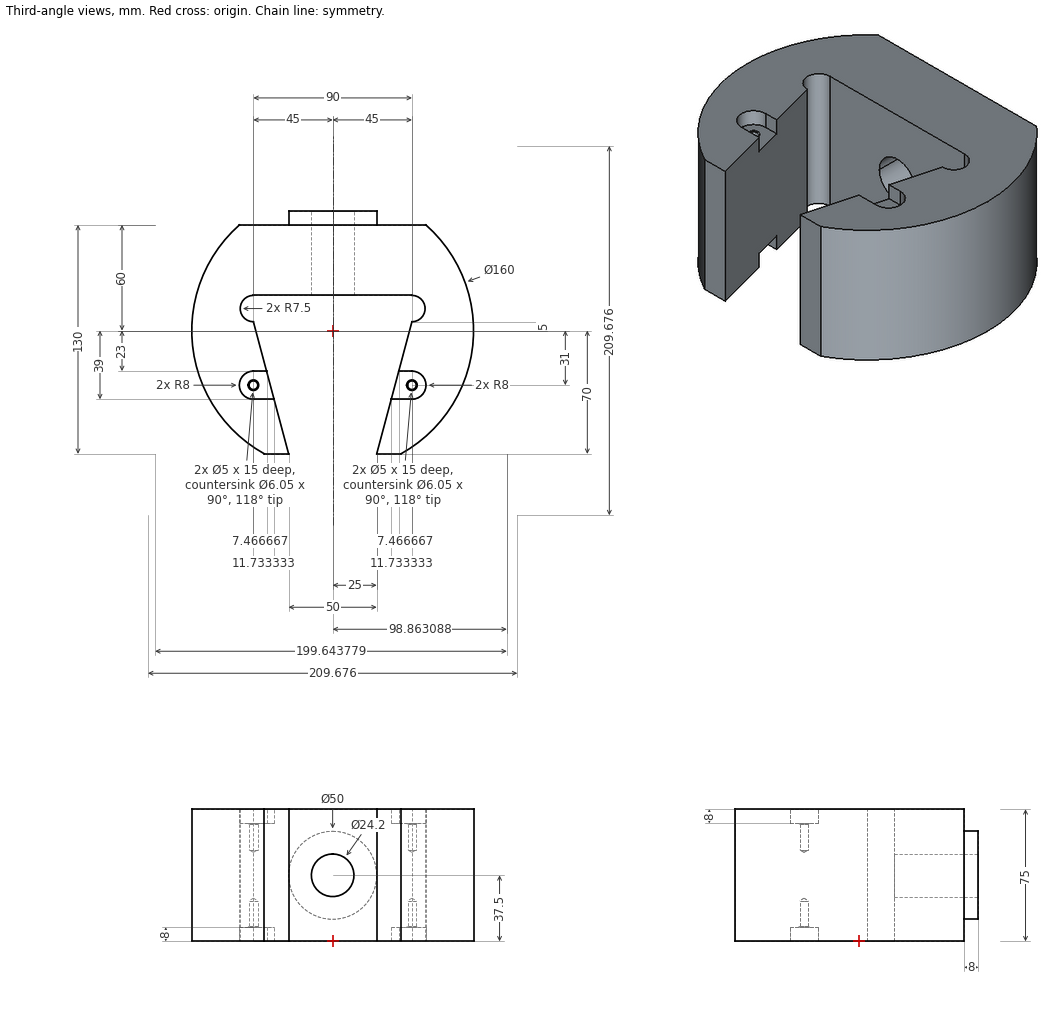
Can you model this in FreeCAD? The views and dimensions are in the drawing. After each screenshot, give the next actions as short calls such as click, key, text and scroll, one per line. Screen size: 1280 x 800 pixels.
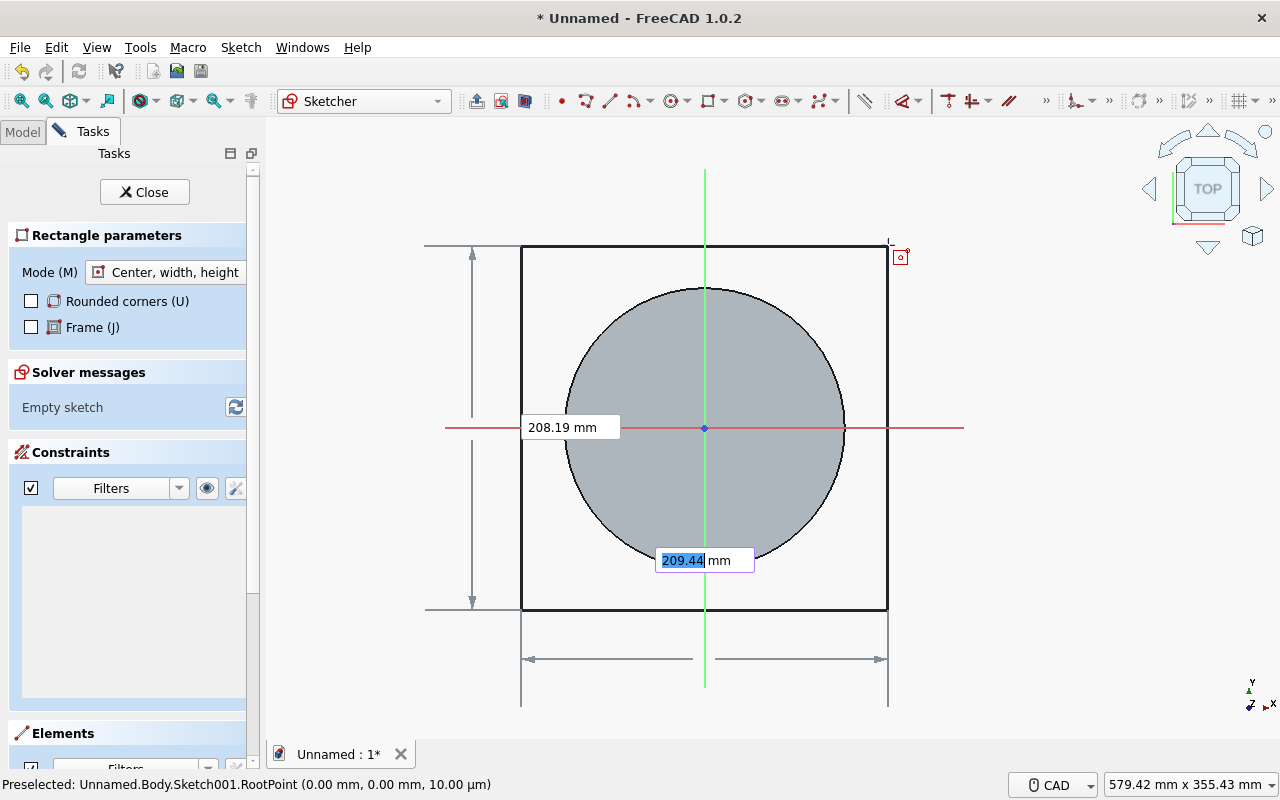
text(209.676)
key(Tab)
text(209.676)
key(Return)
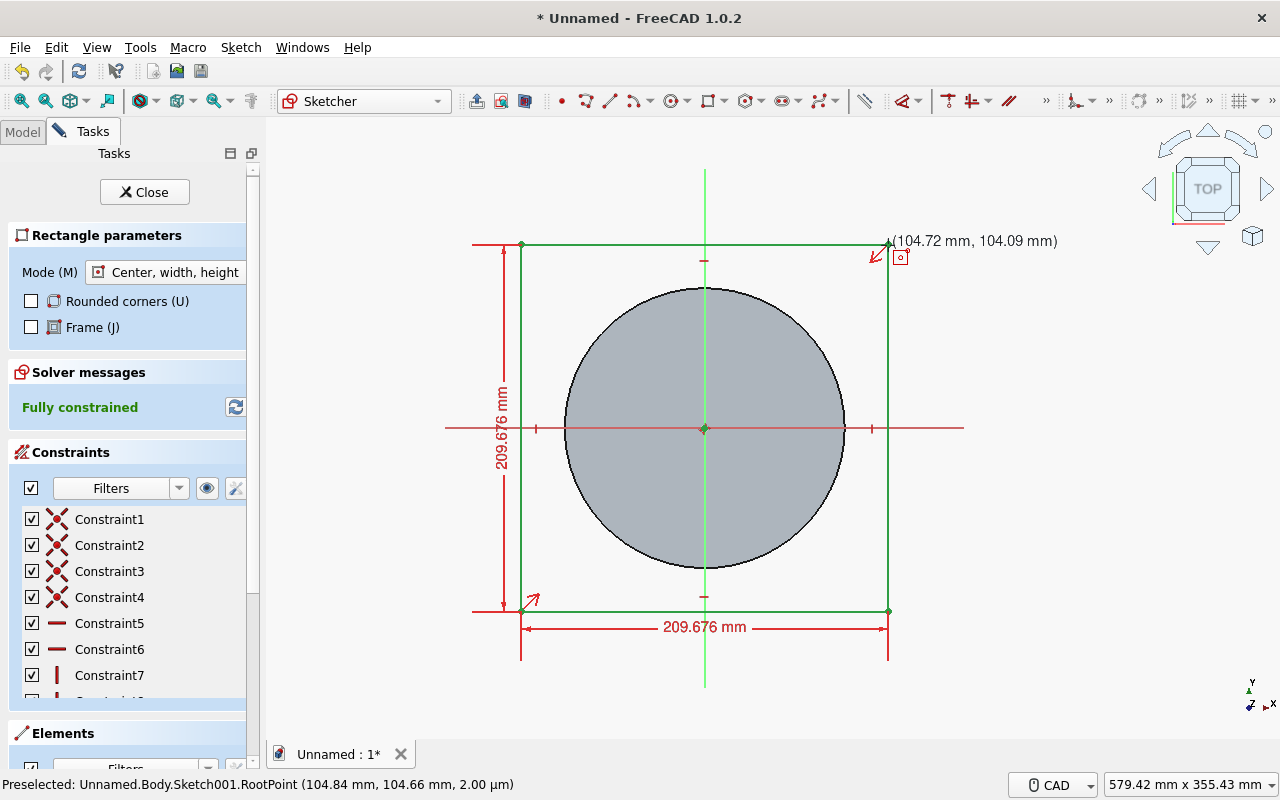
key(g)
key(r)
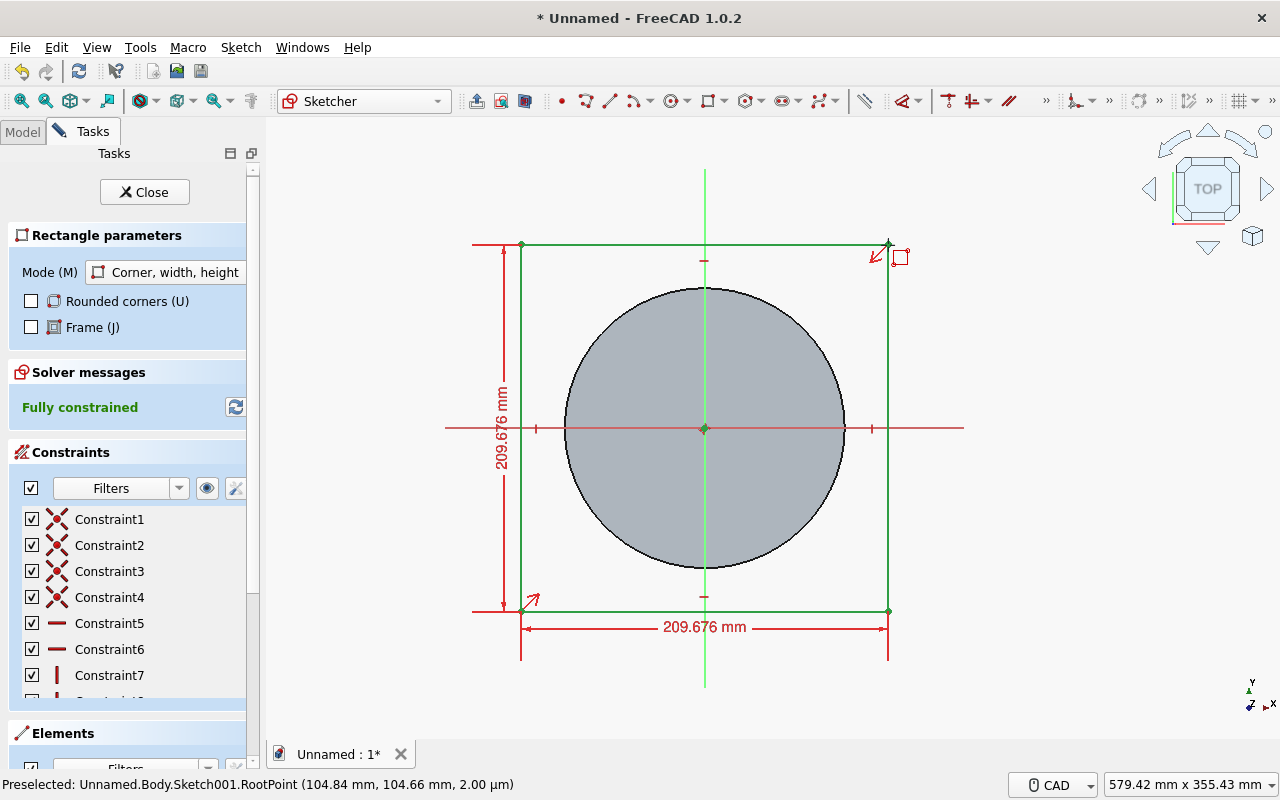
scroll(528, 323, up, 5)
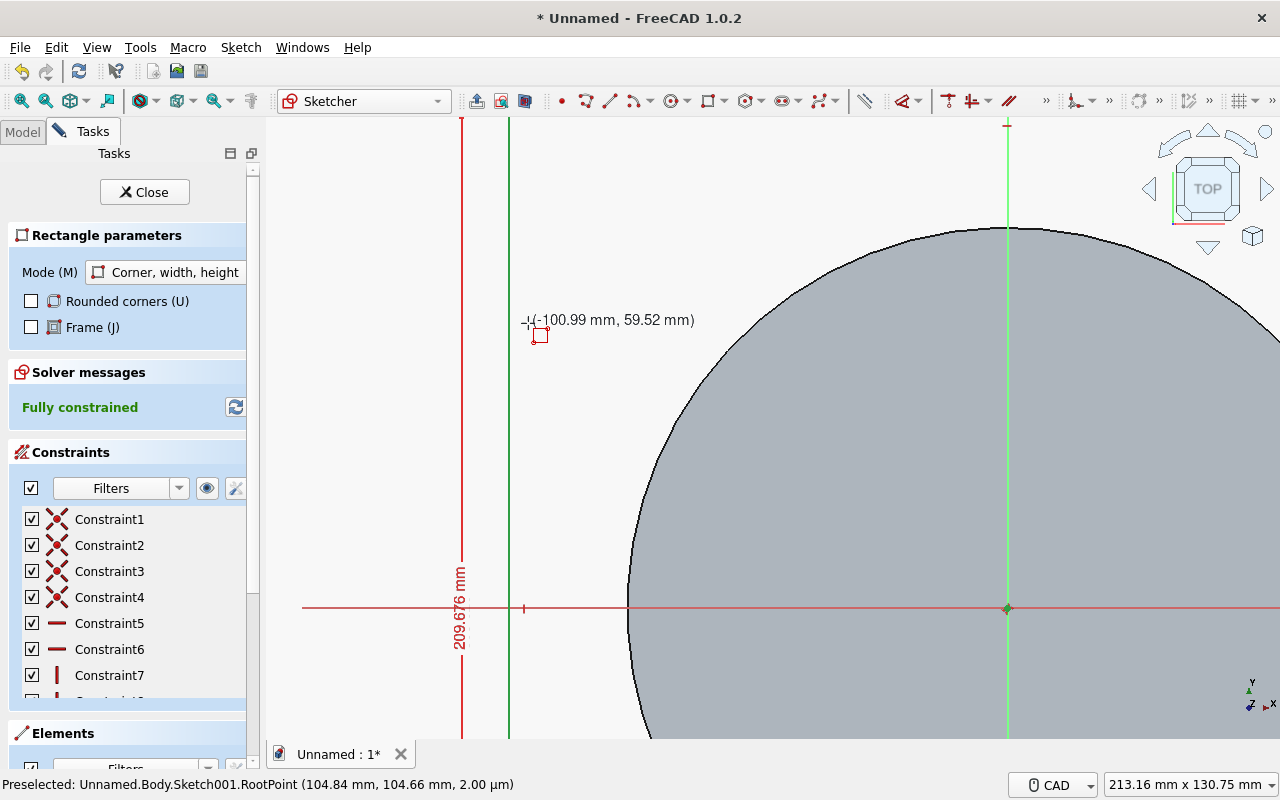
click(529, 323)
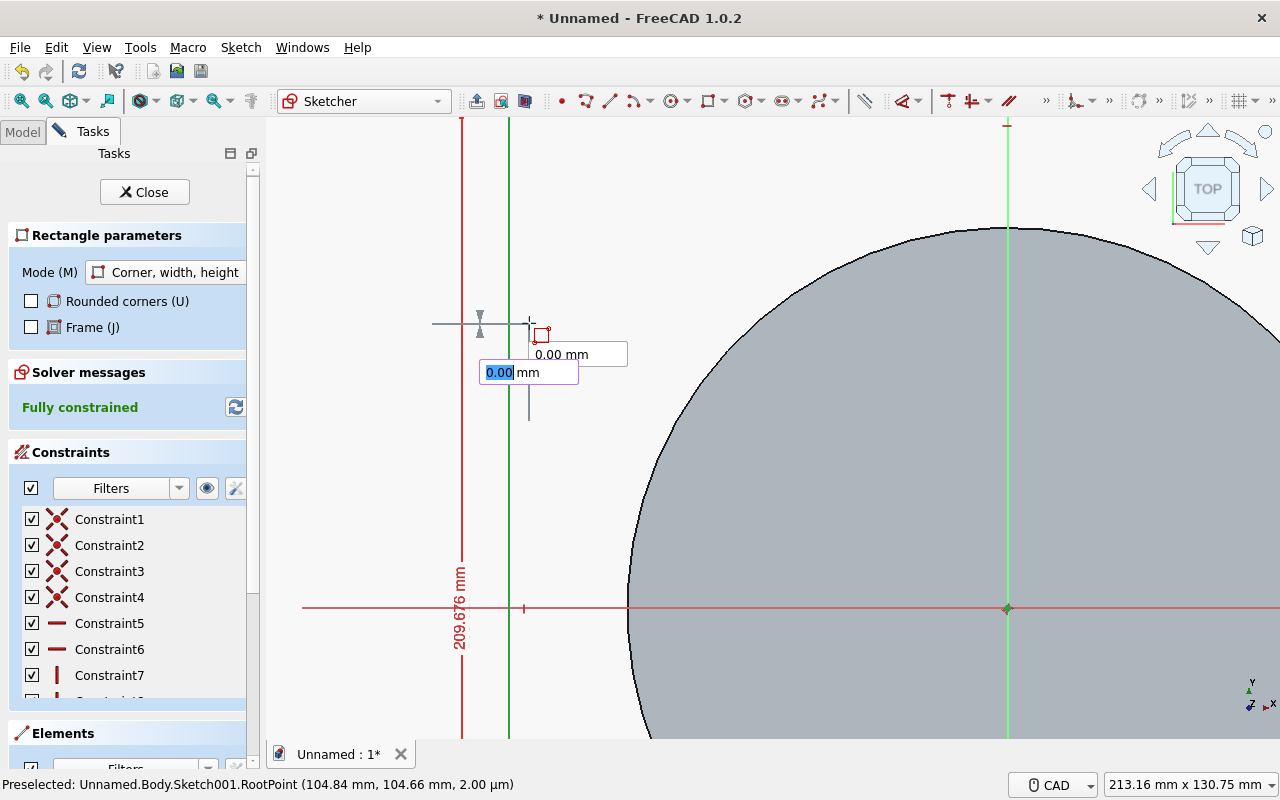
scroll(528, 323, down, 5)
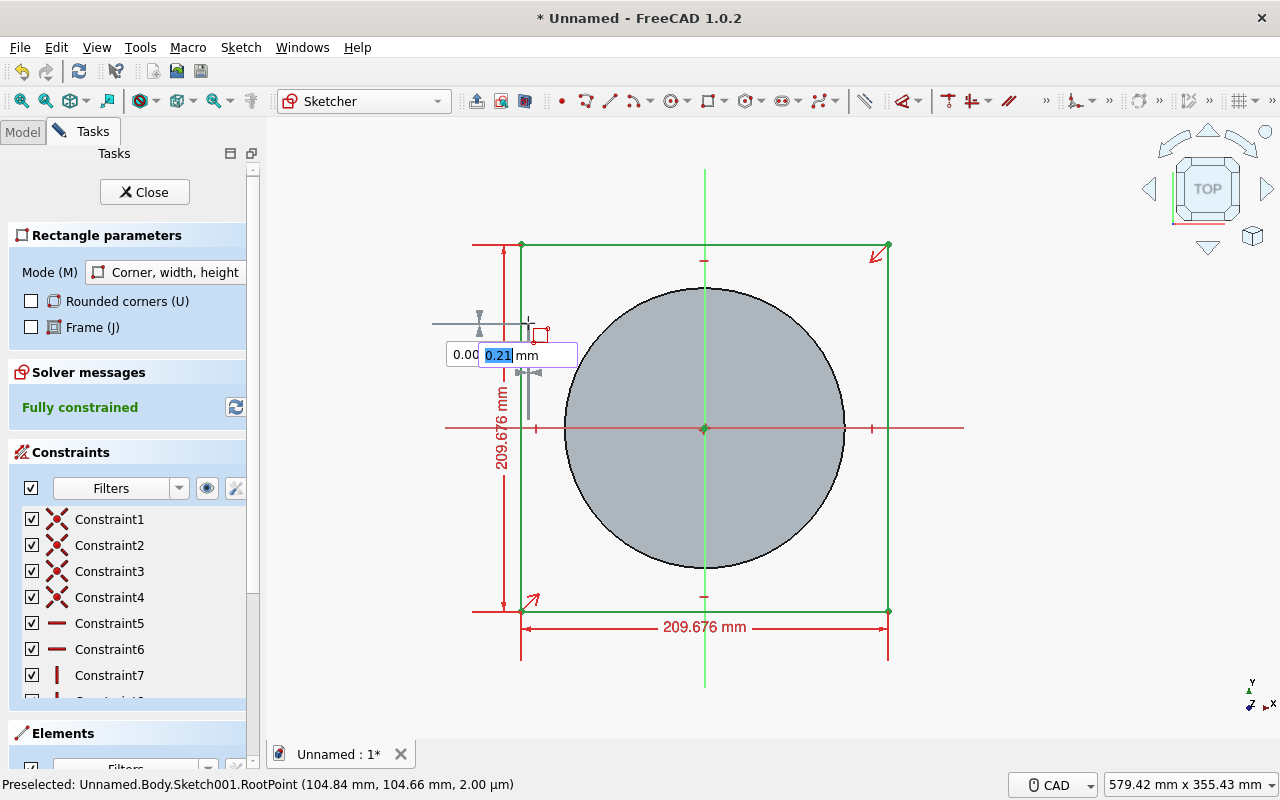
scroll(878, 551, up, 3)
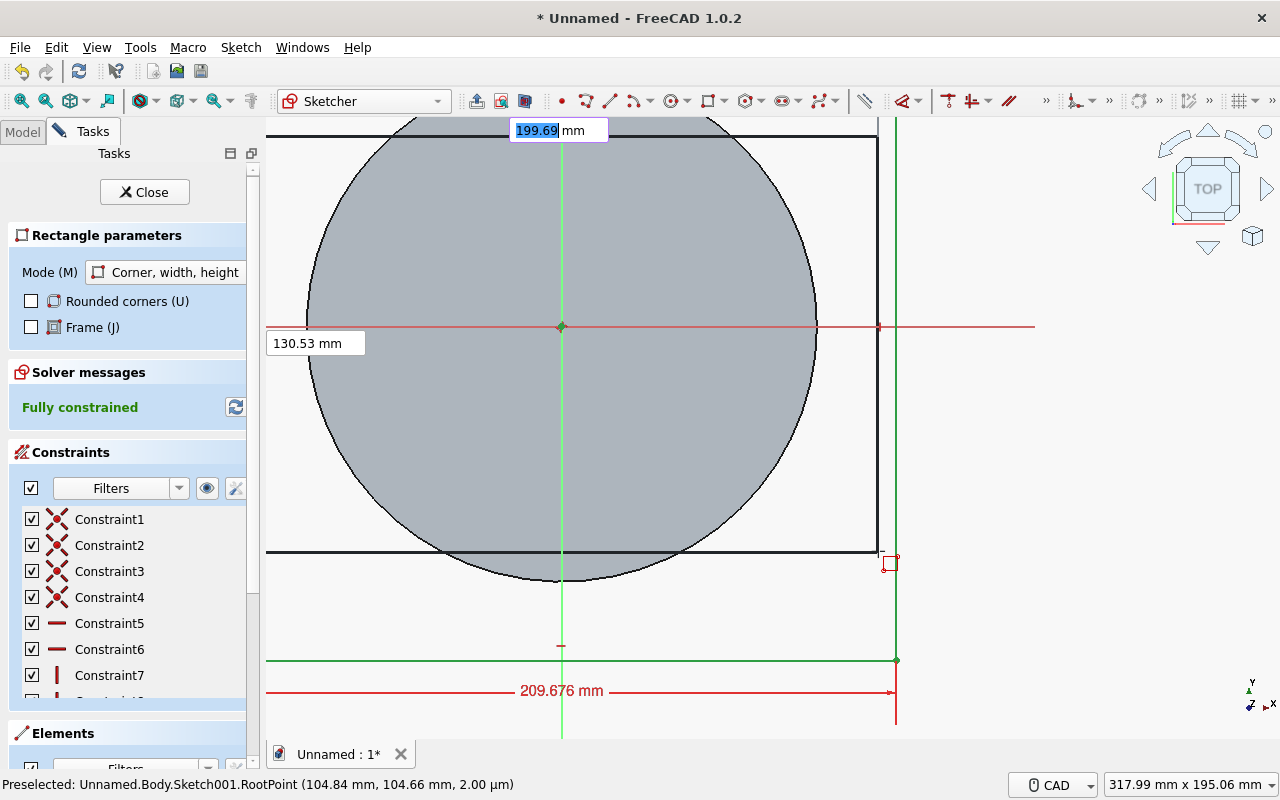
click(877, 550)
key(Escape)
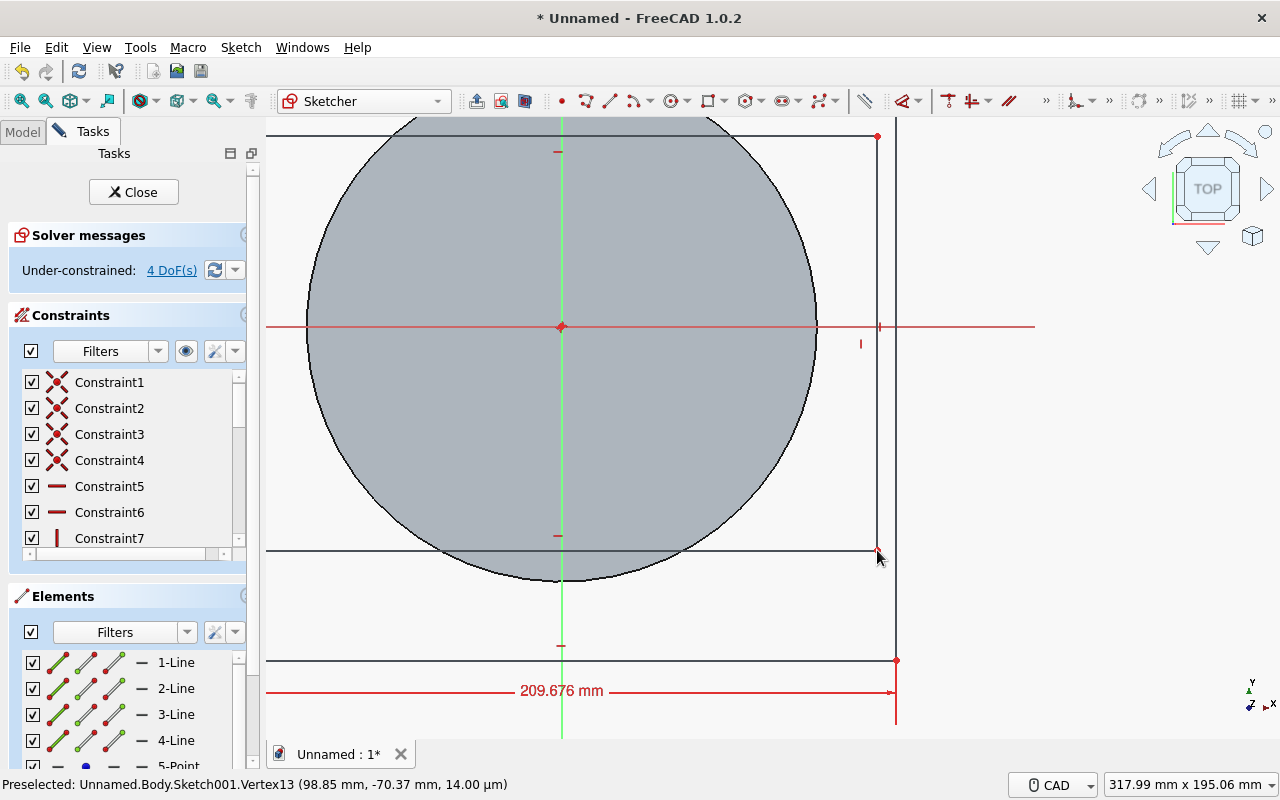
click(902, 102)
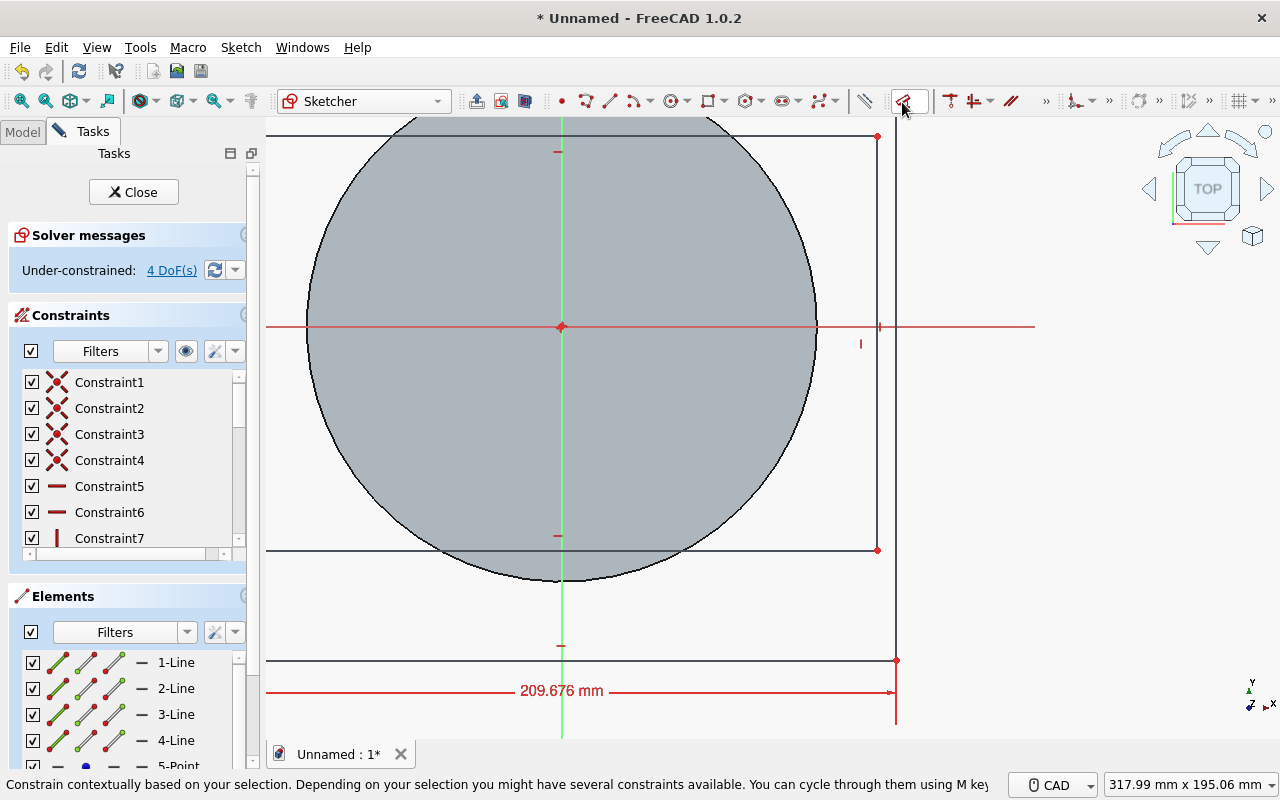
scroll(878, 551, down, 3)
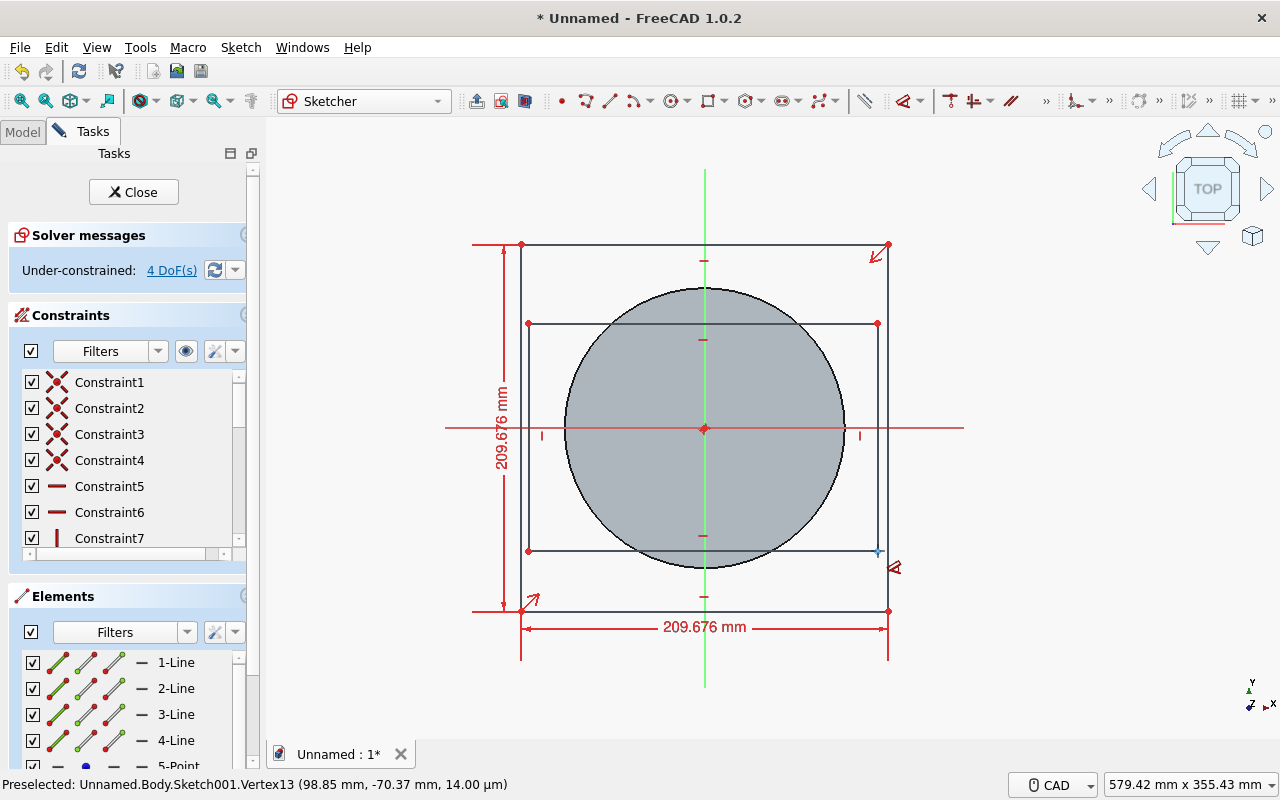
scroll(529, 392, up, 4)